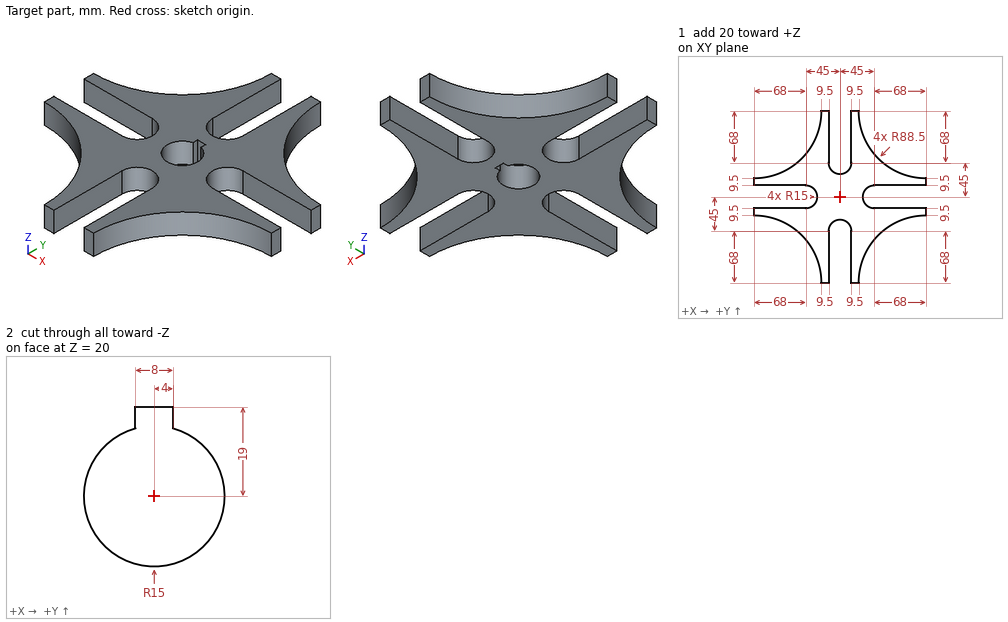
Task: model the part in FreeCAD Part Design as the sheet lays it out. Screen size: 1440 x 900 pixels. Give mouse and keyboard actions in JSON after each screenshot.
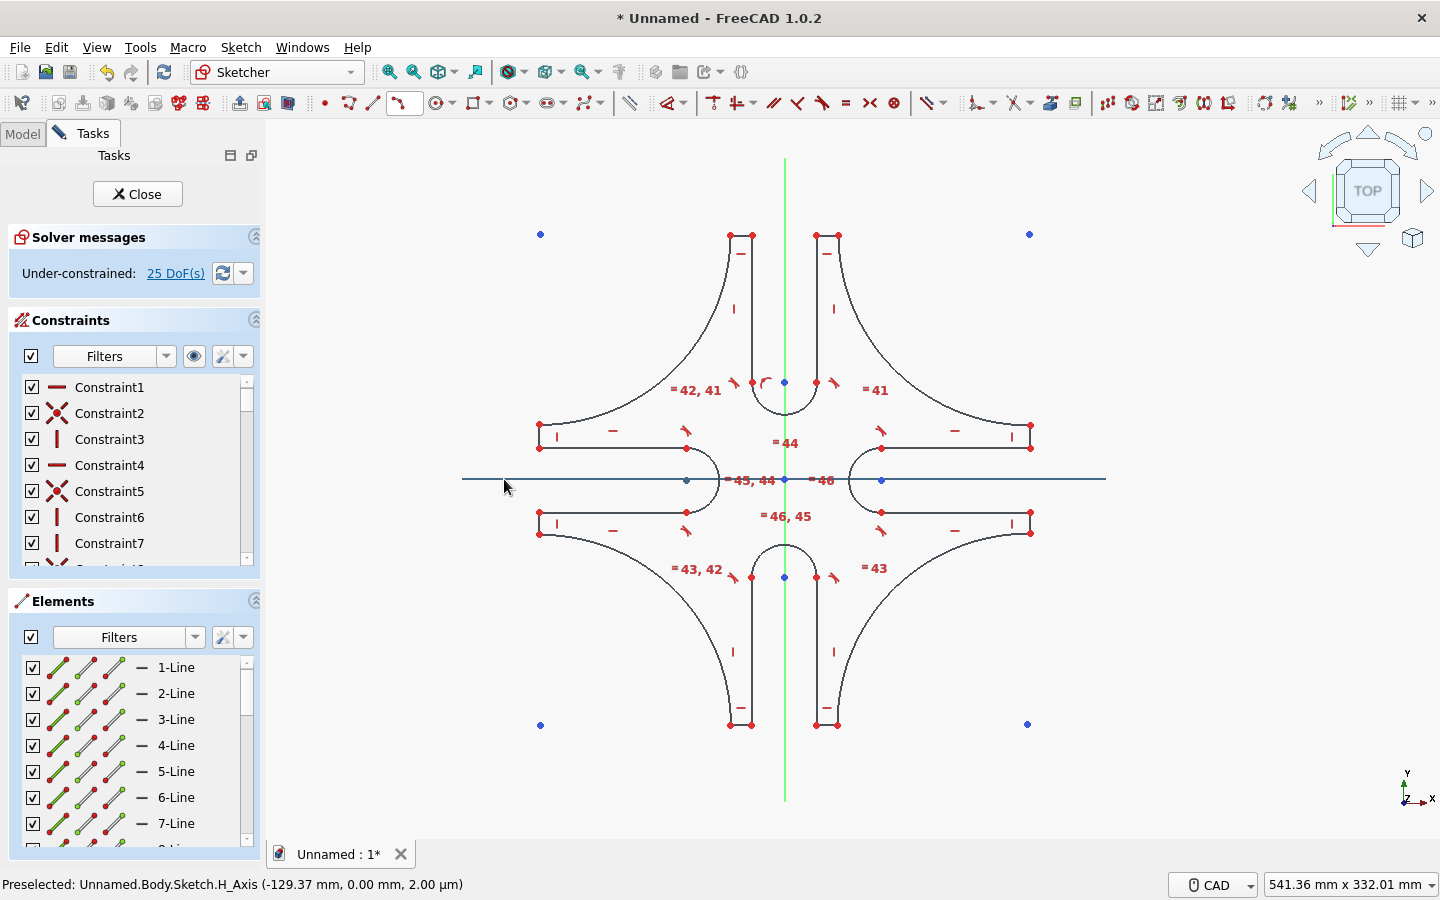
{"action": "left_click", "coordinate": [714, 104]}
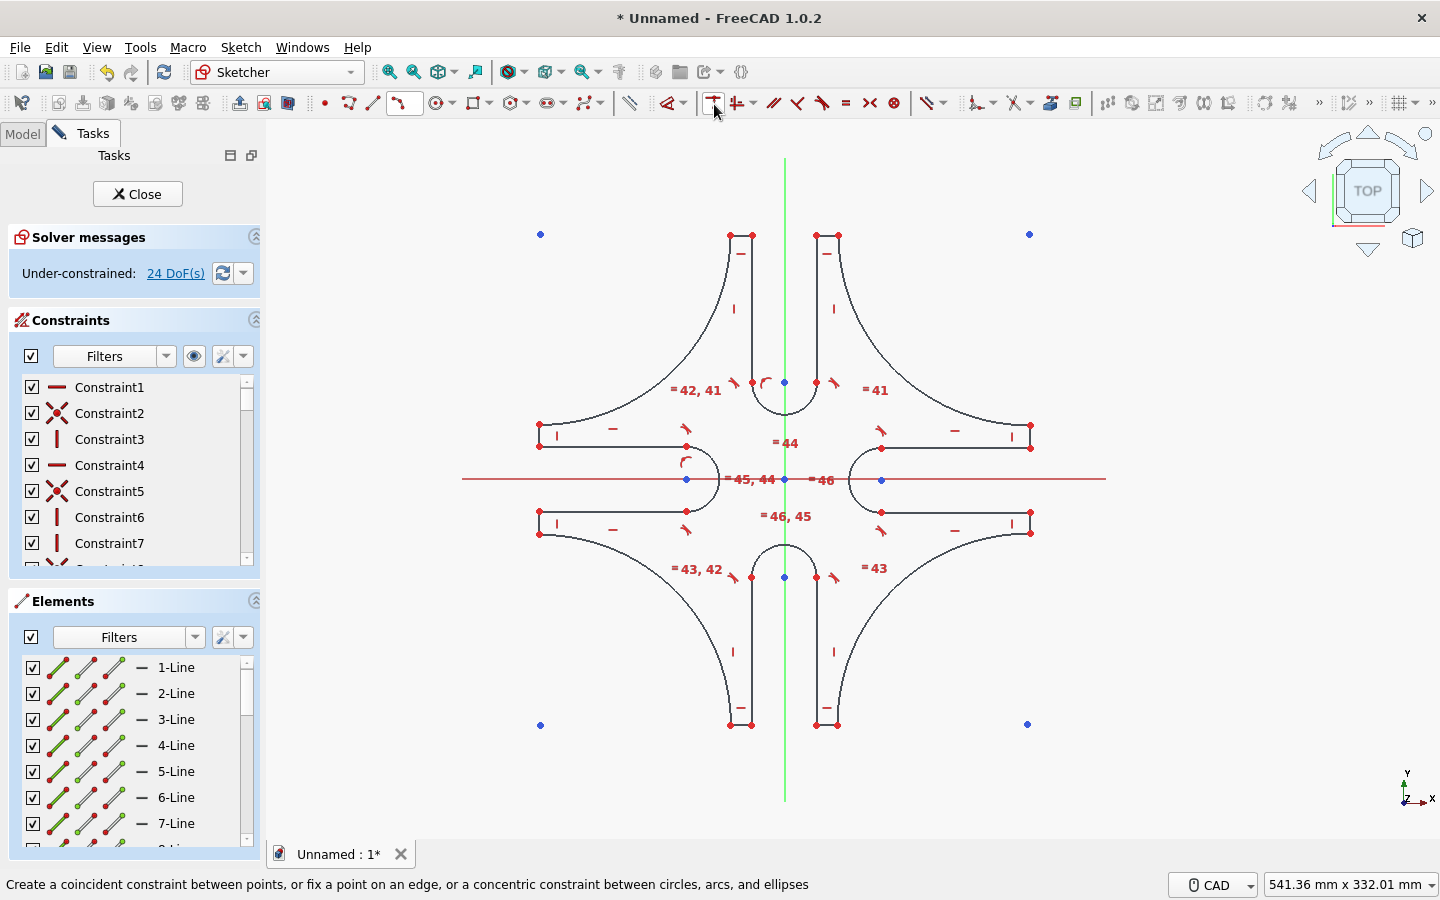
{"action": "left_click", "coordinate": [784, 577]}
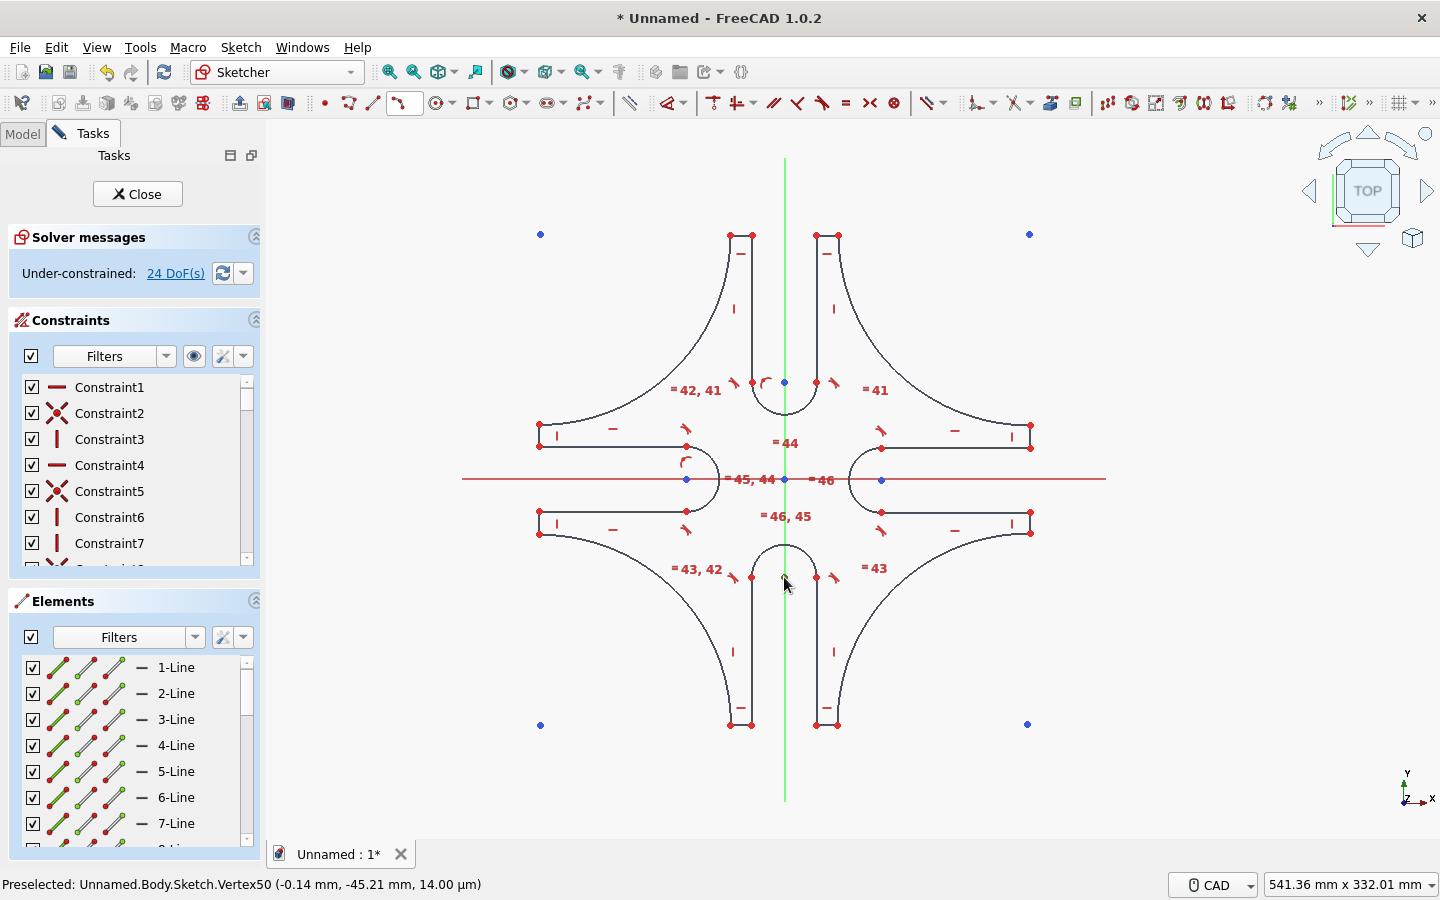
{"action": "left_click", "coordinate": [785, 764]}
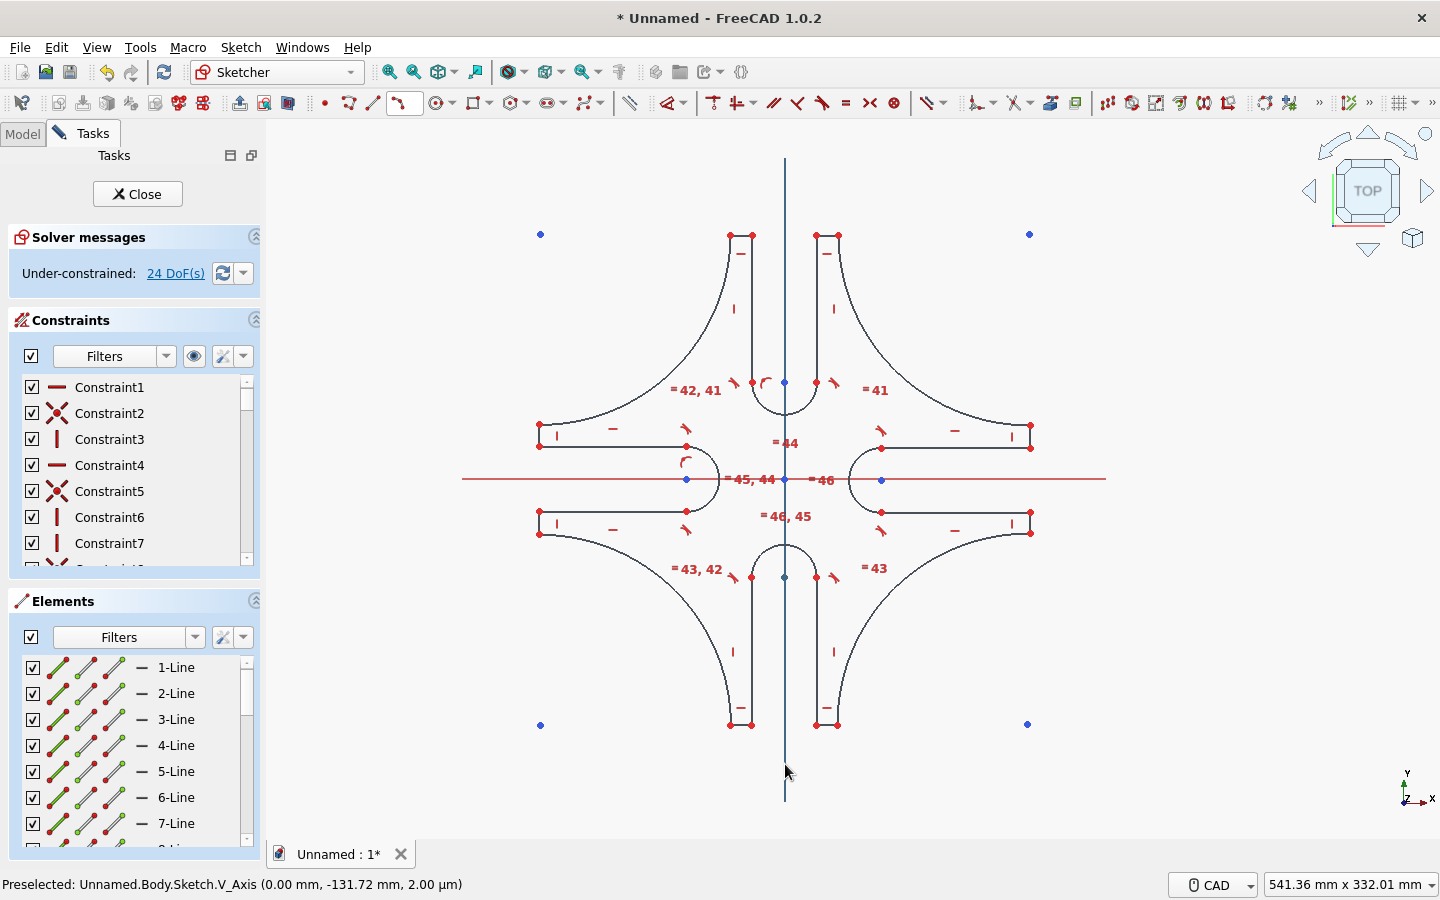
{"action": "left_click", "coordinate": [714, 104]}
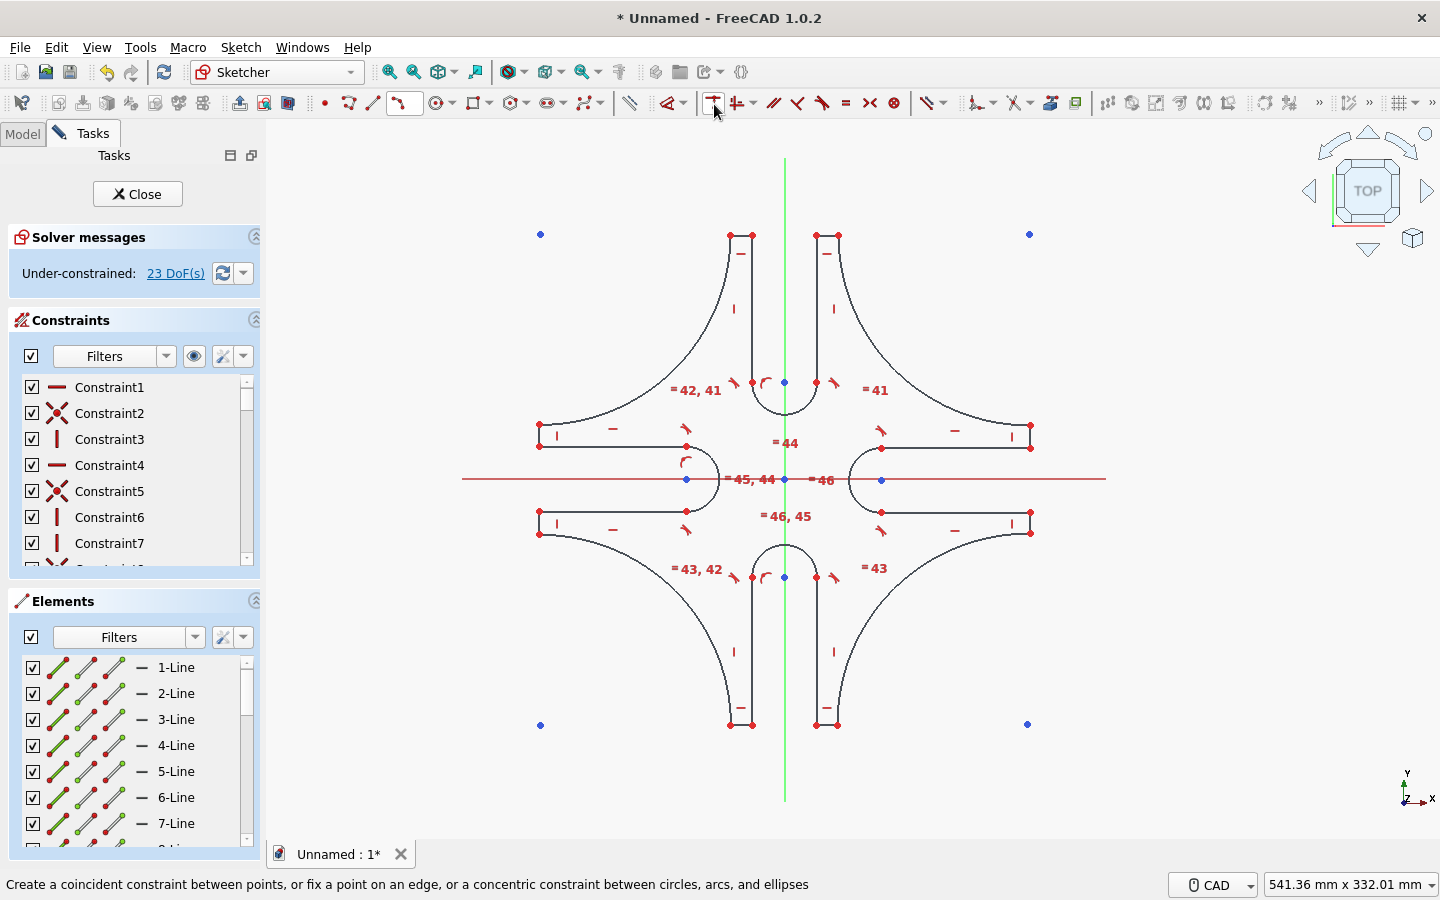
{"action": "left_click", "coordinate": [882, 480]}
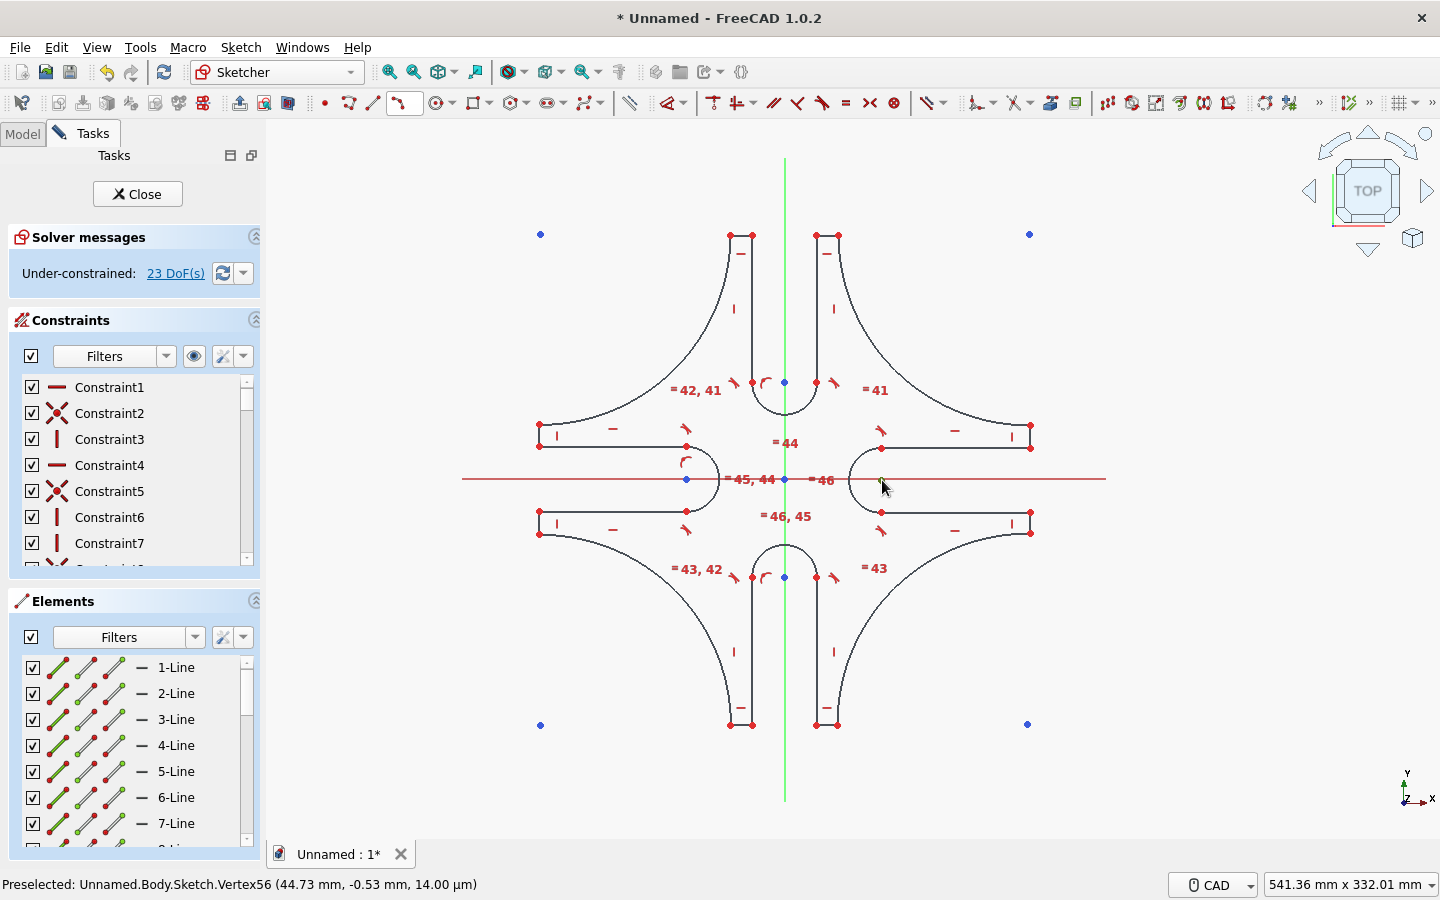
{"action": "left_click", "coordinate": [504, 479]}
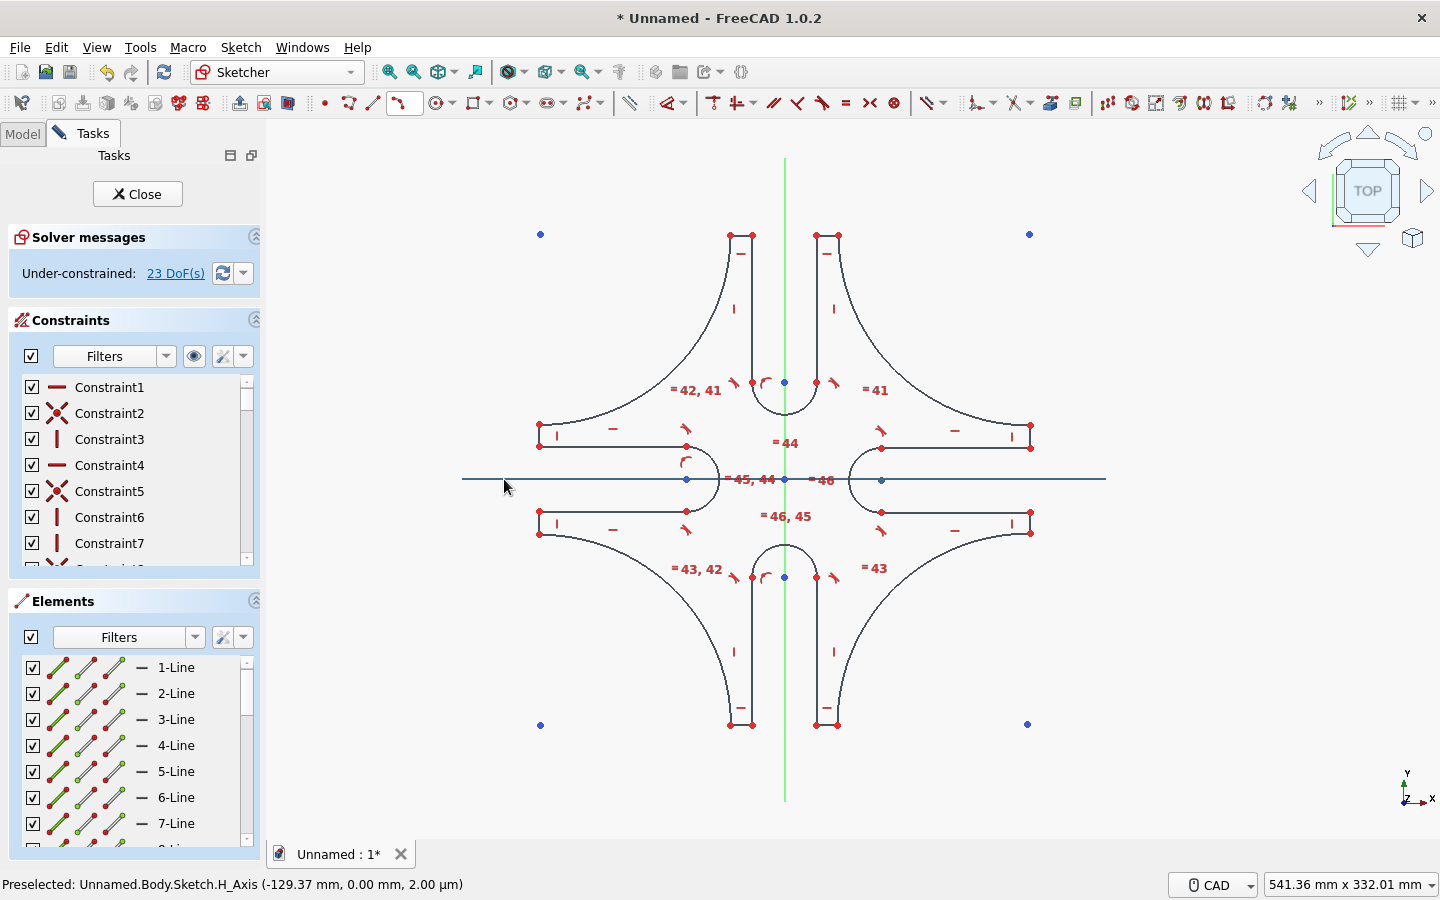
{"action": "left_click", "coordinate": [714, 104]}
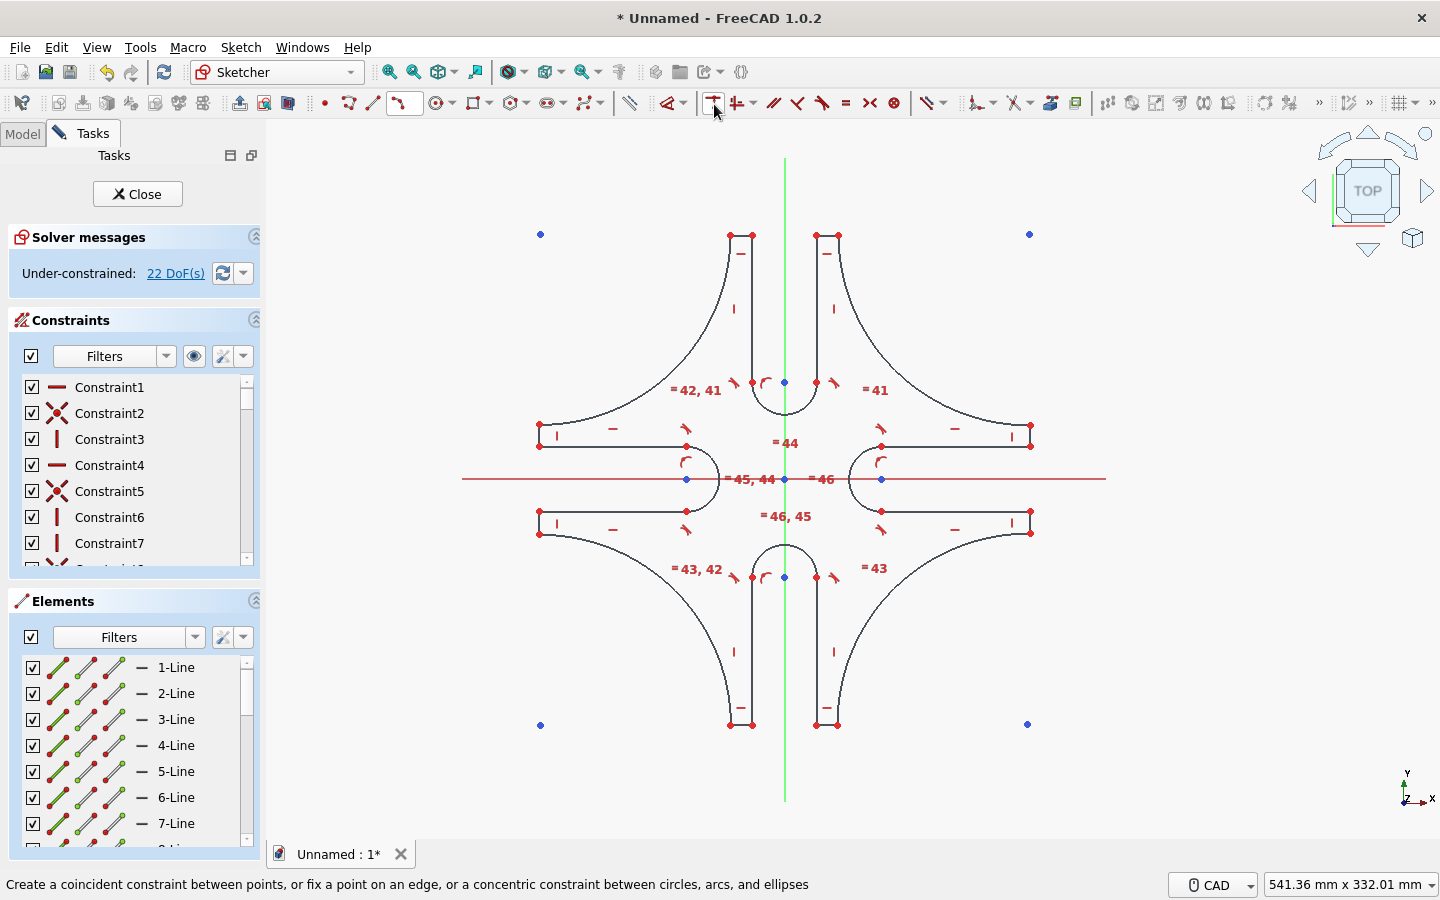
{"action": "left_click", "coordinate": [668, 104]}